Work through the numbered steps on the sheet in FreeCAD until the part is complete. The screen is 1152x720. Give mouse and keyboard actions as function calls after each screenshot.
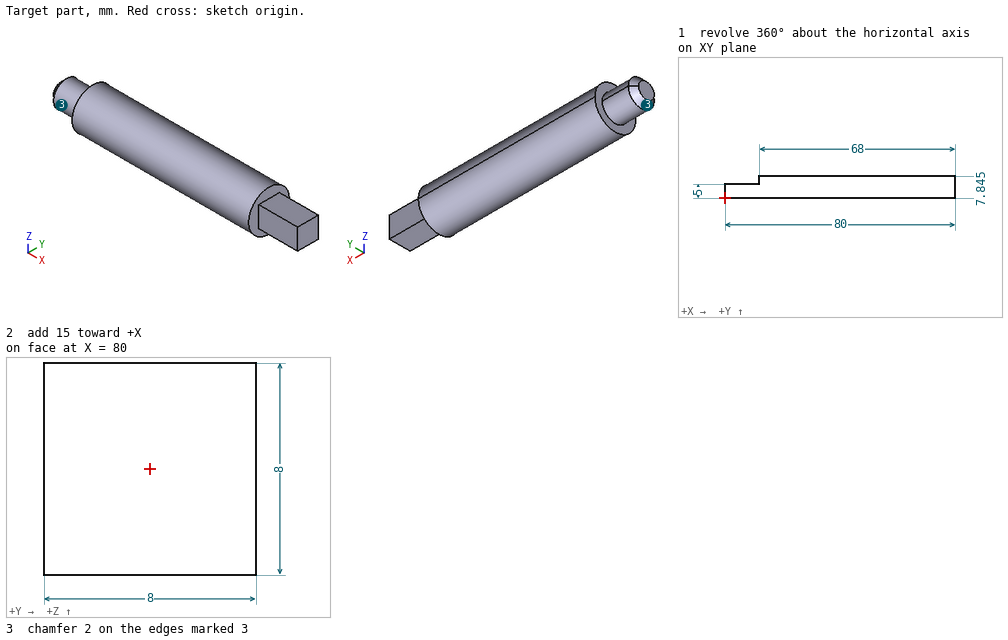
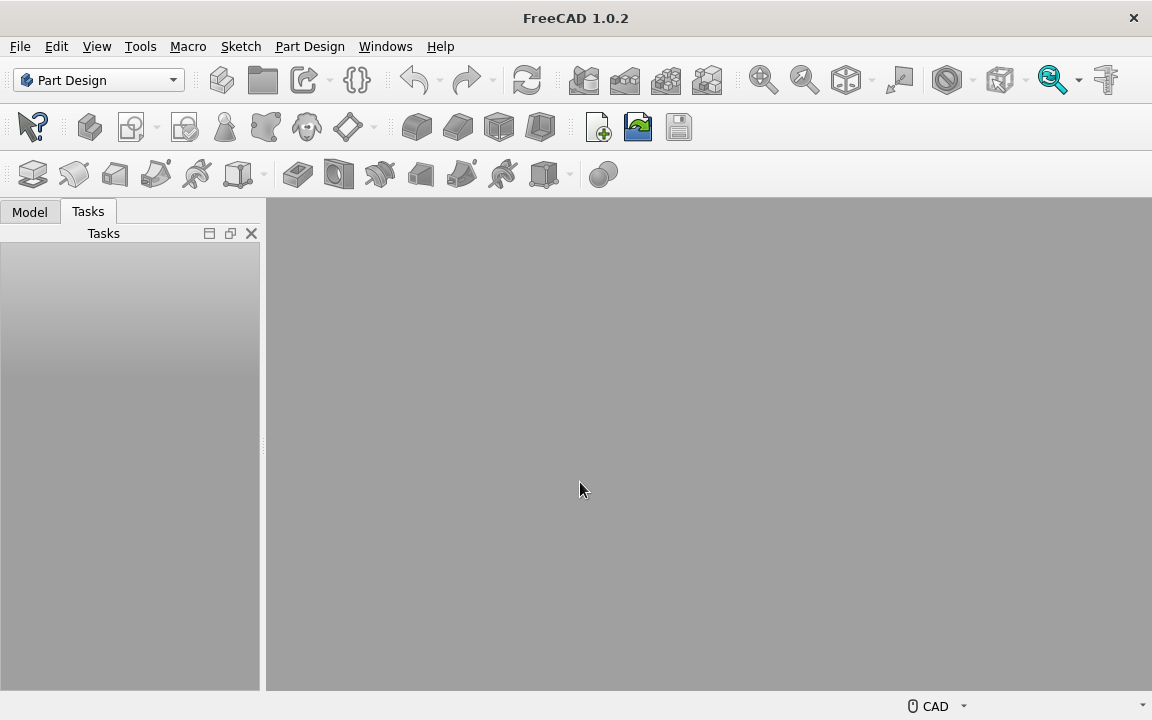
click(597, 128)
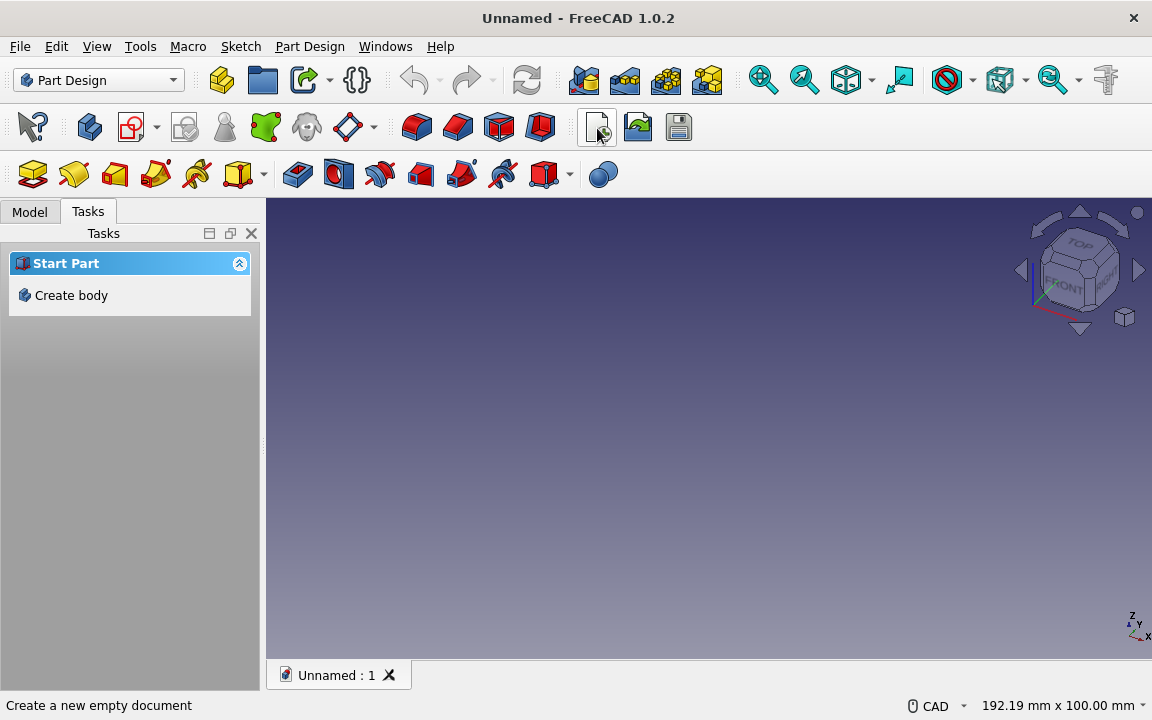
click(130, 128)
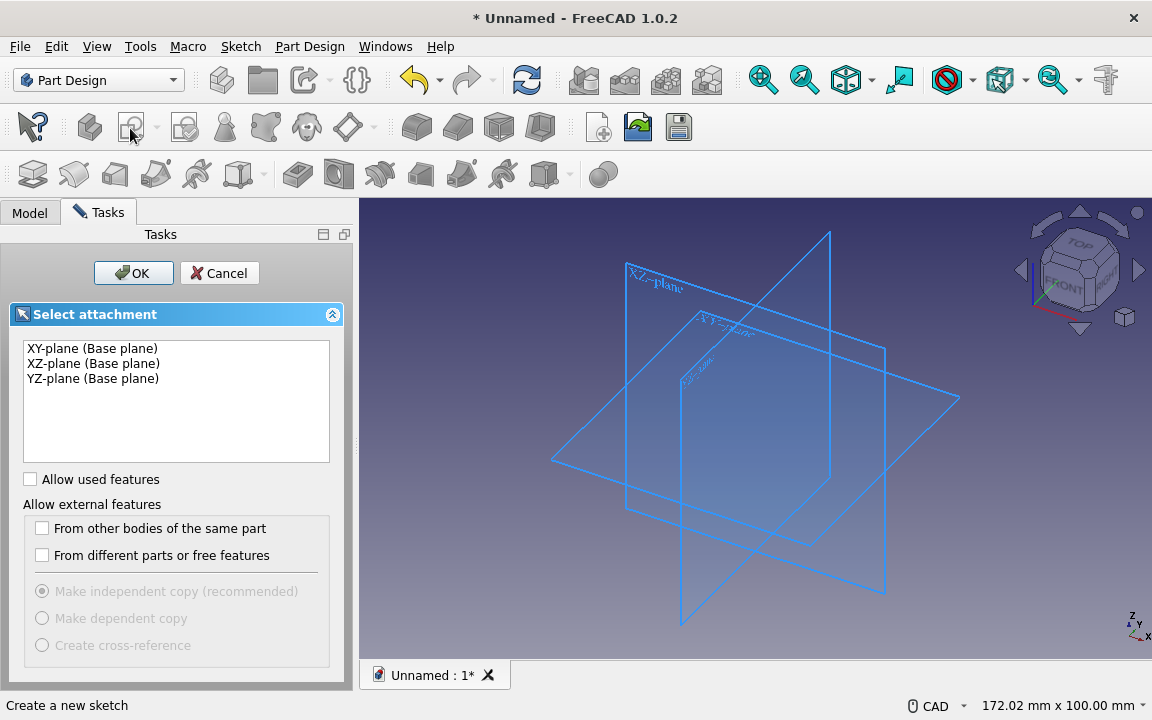
click(84, 348)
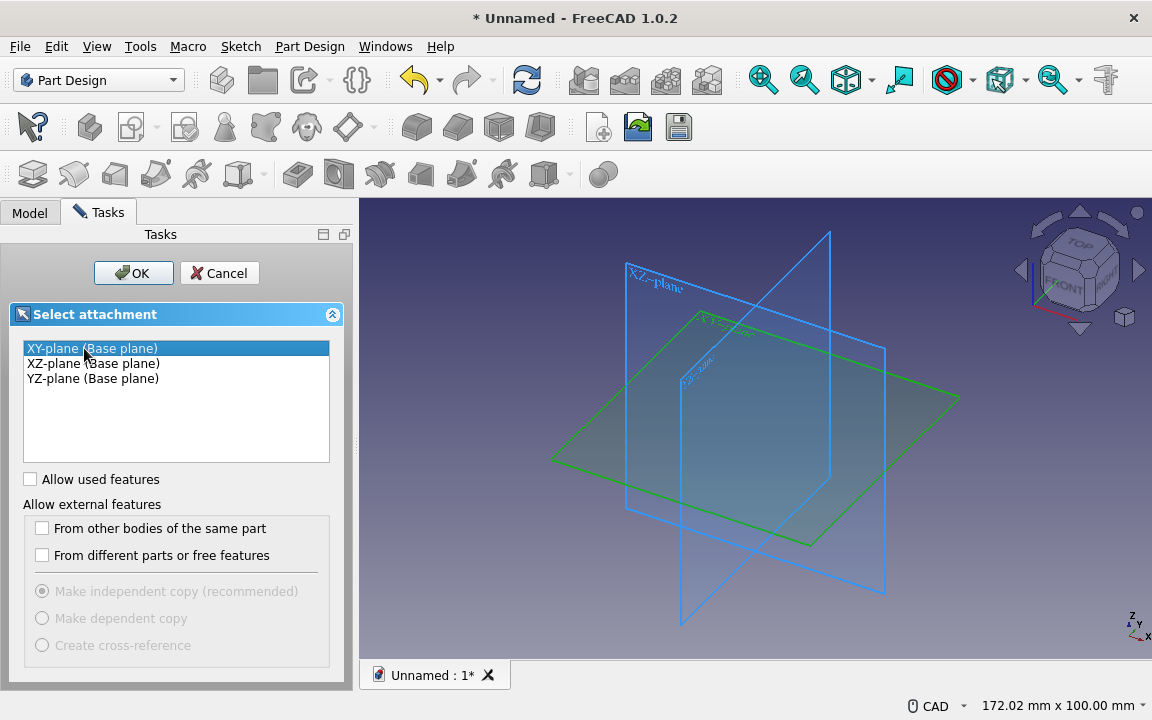
click(134, 273)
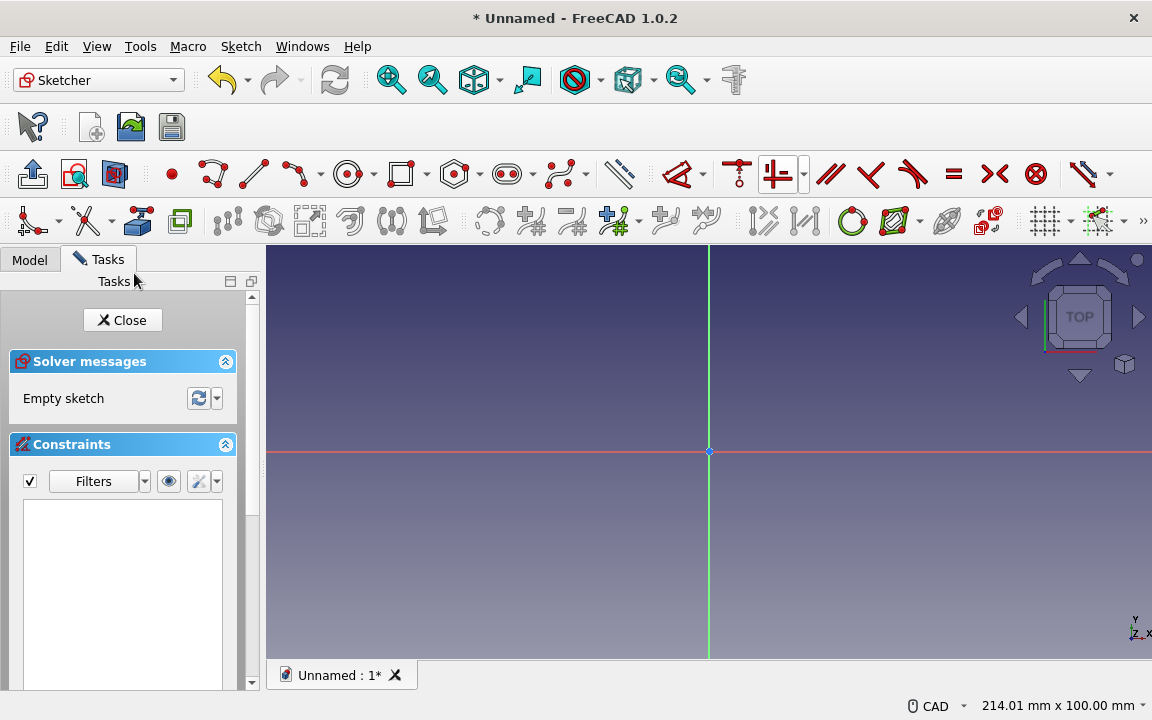
scroll(294, 525, down, 1)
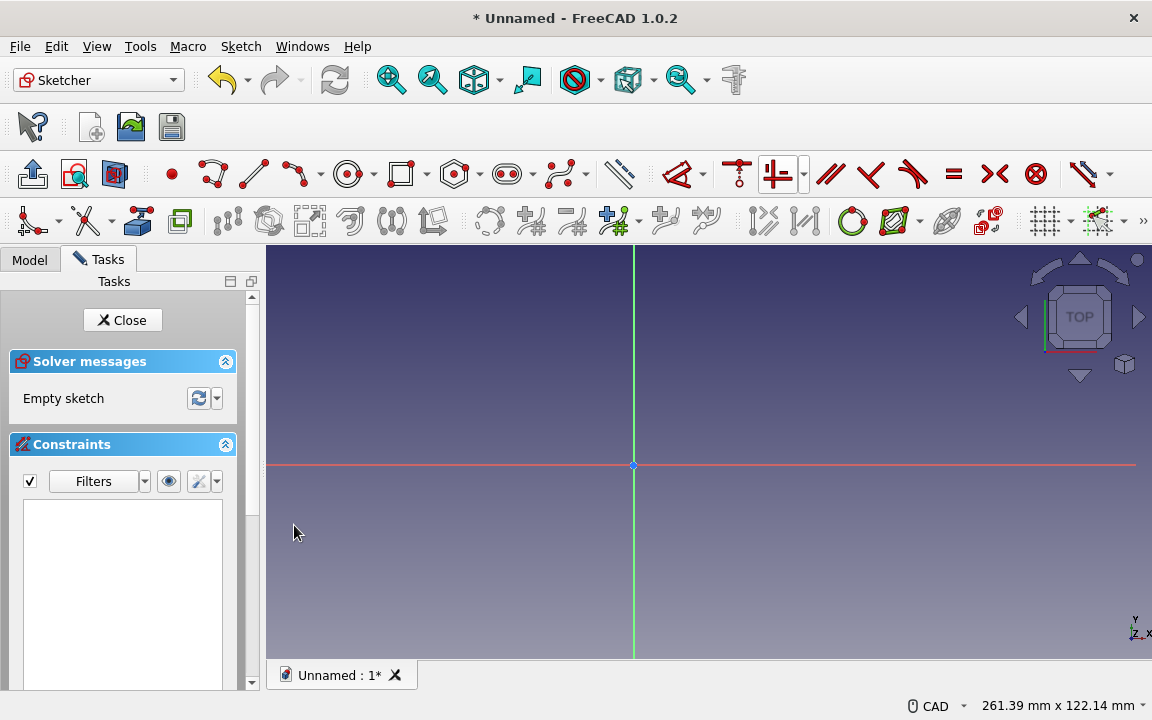
scroll(926, 452, up, 3)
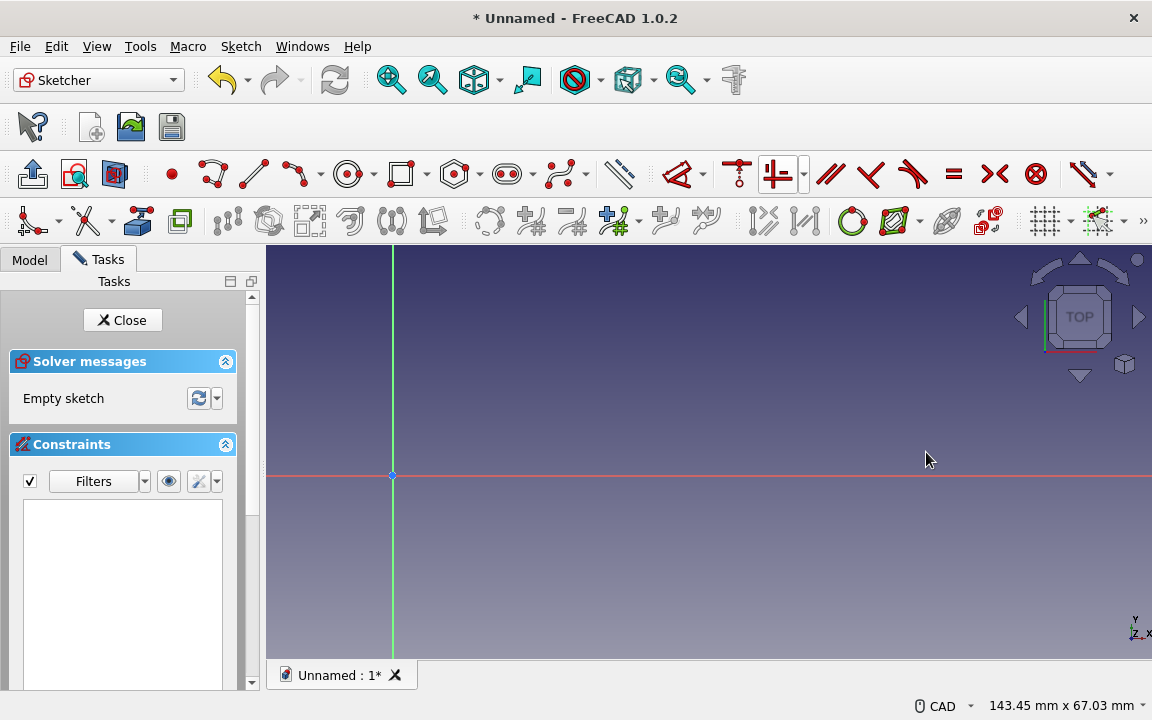
click(213, 174)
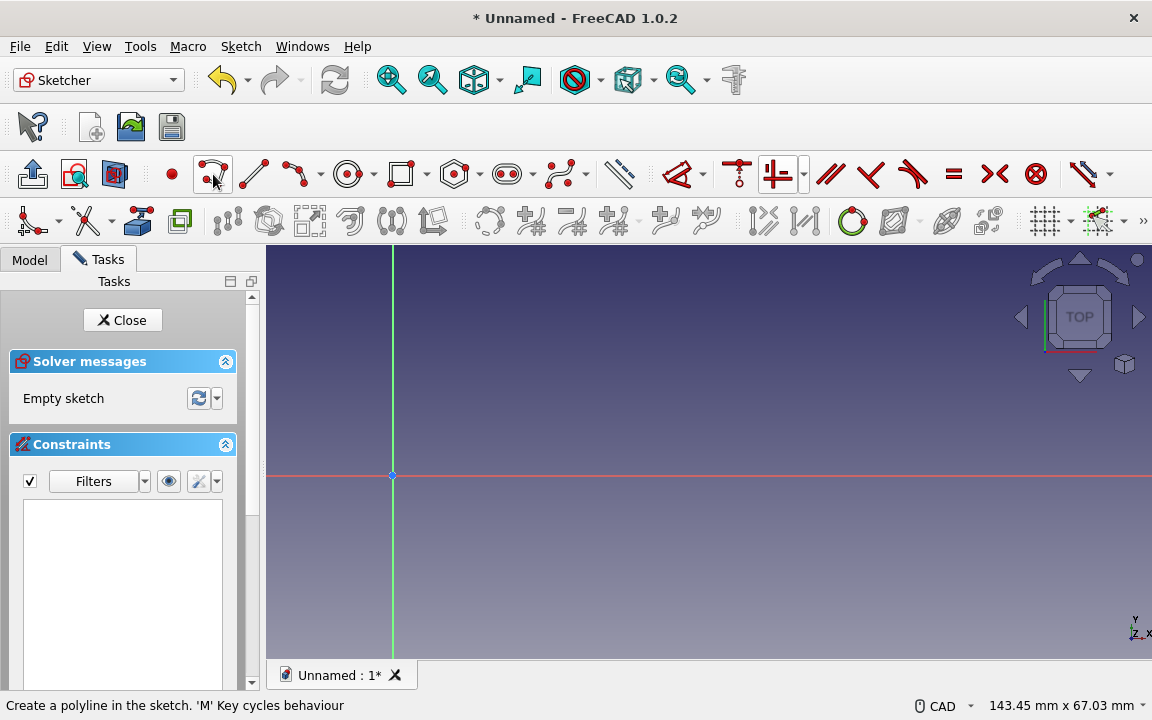
click(393, 476)
click(887, 467)
click(887, 427)
click(467, 427)
click(467, 445)
click(402, 445)
click(393, 476)
key(Escape)
key(Escape)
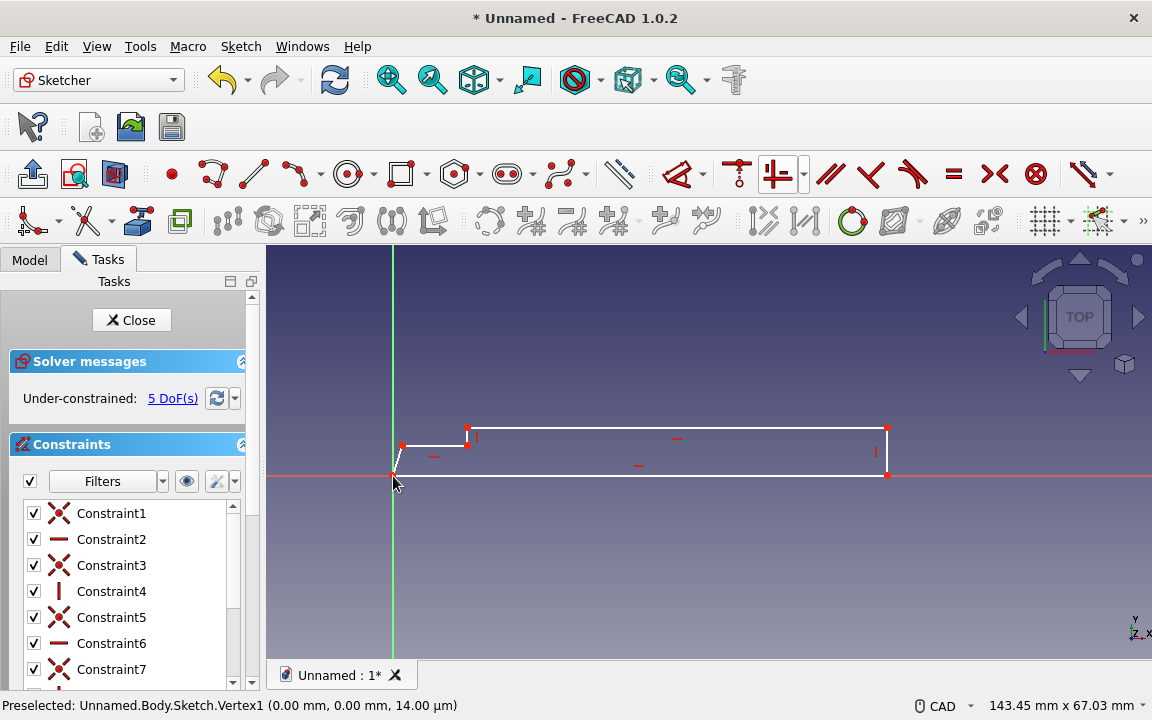
click(397, 464)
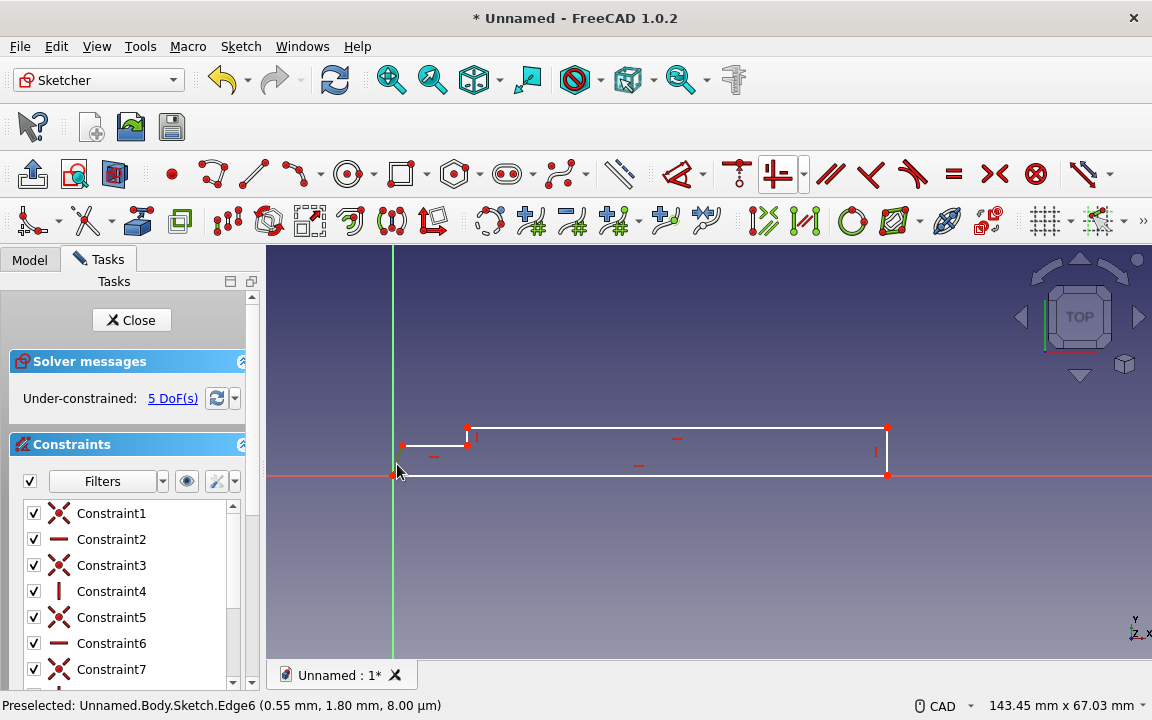
click(804, 174)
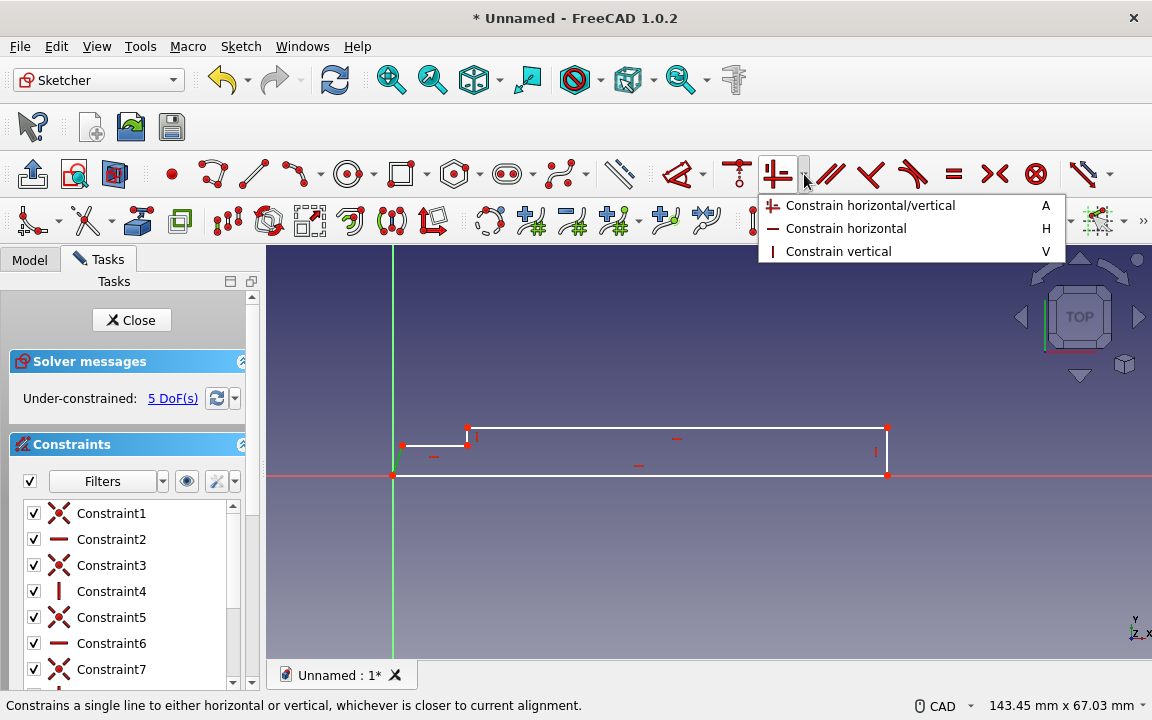
click(912, 252)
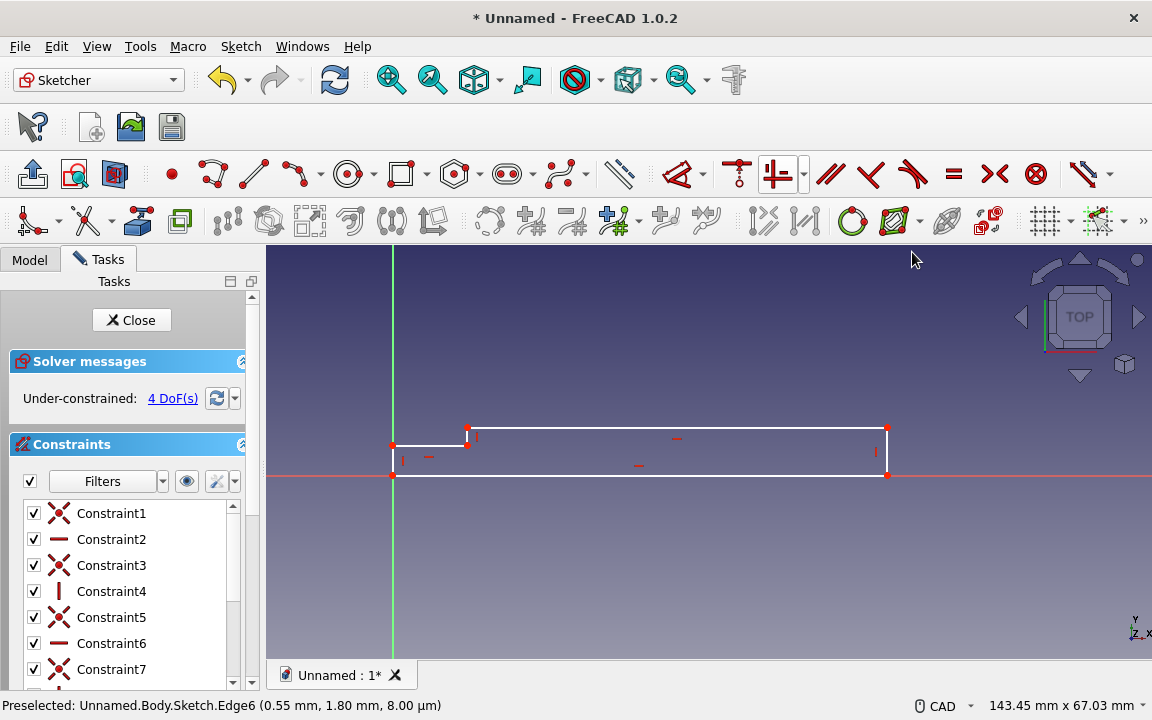
click(676, 174)